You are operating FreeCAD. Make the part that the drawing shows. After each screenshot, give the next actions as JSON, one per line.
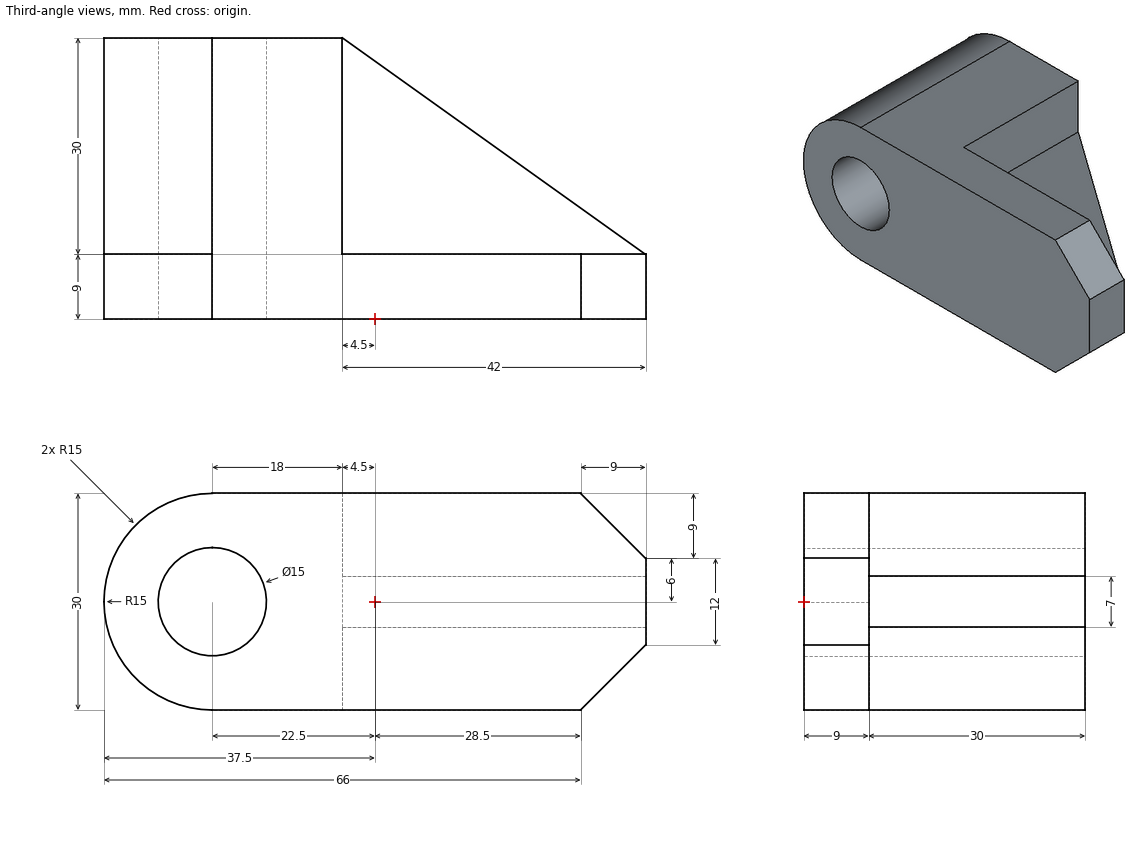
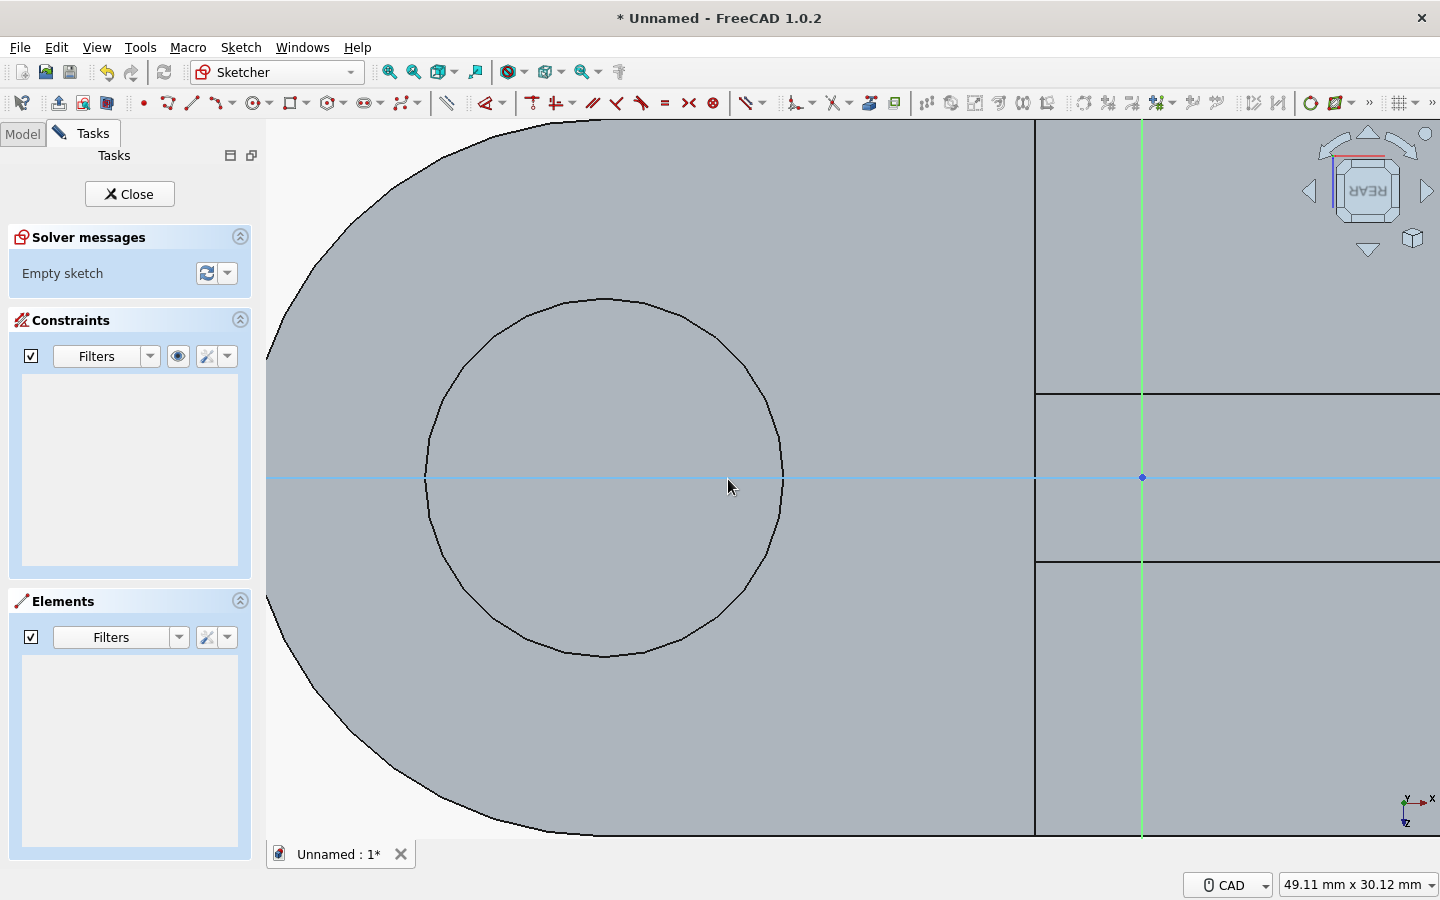
{"action": "left_click", "coordinate": [254, 104]}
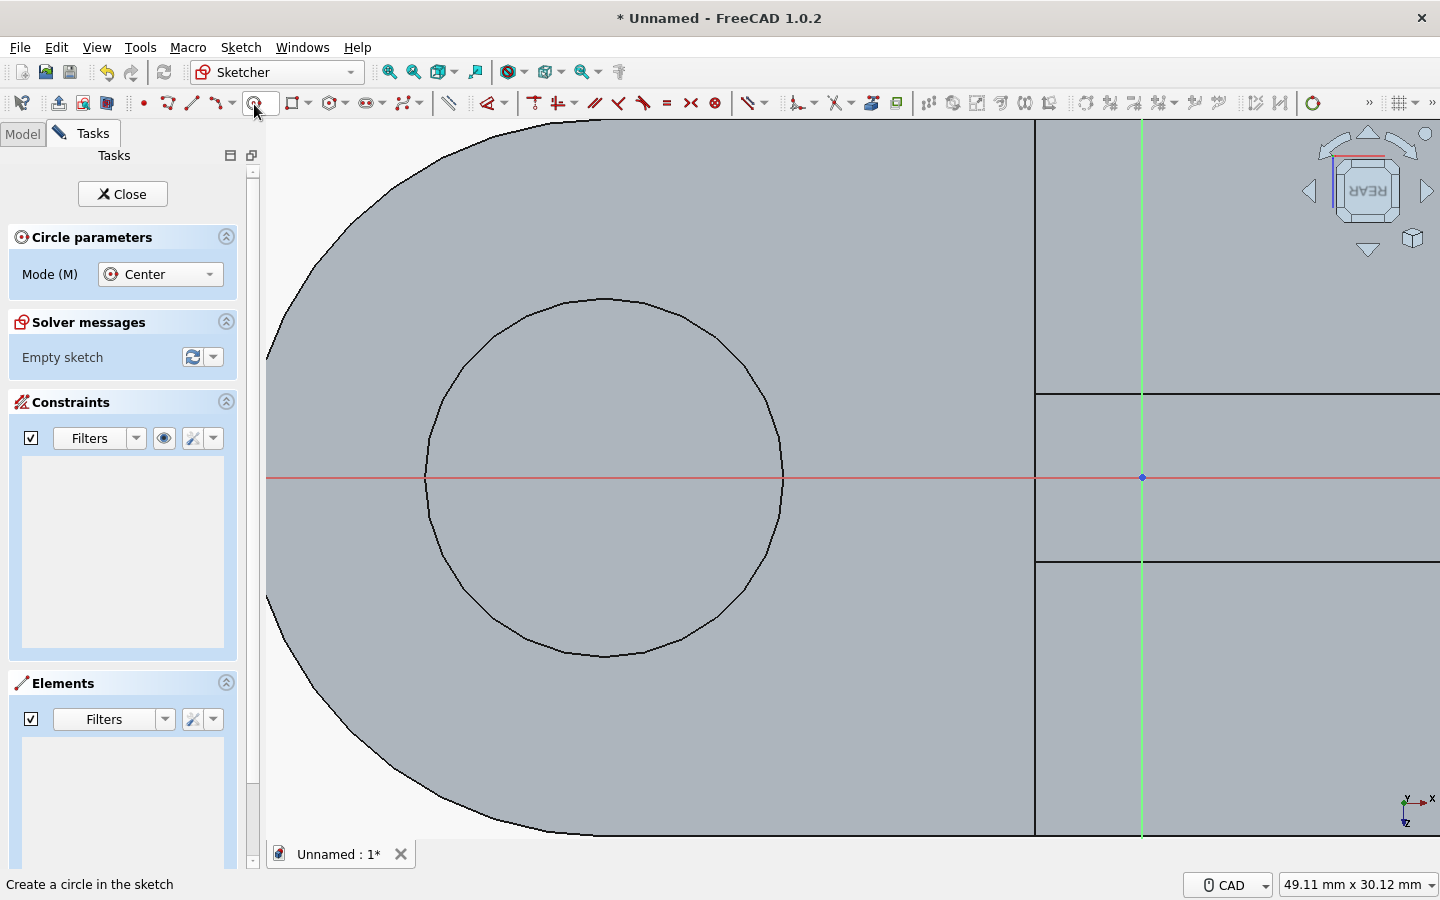
{"action": "left_click", "coordinate": [604, 478]}
{"action": "left_click", "coordinate": [731, 351]}
{"action": "key", "text": "Escape"}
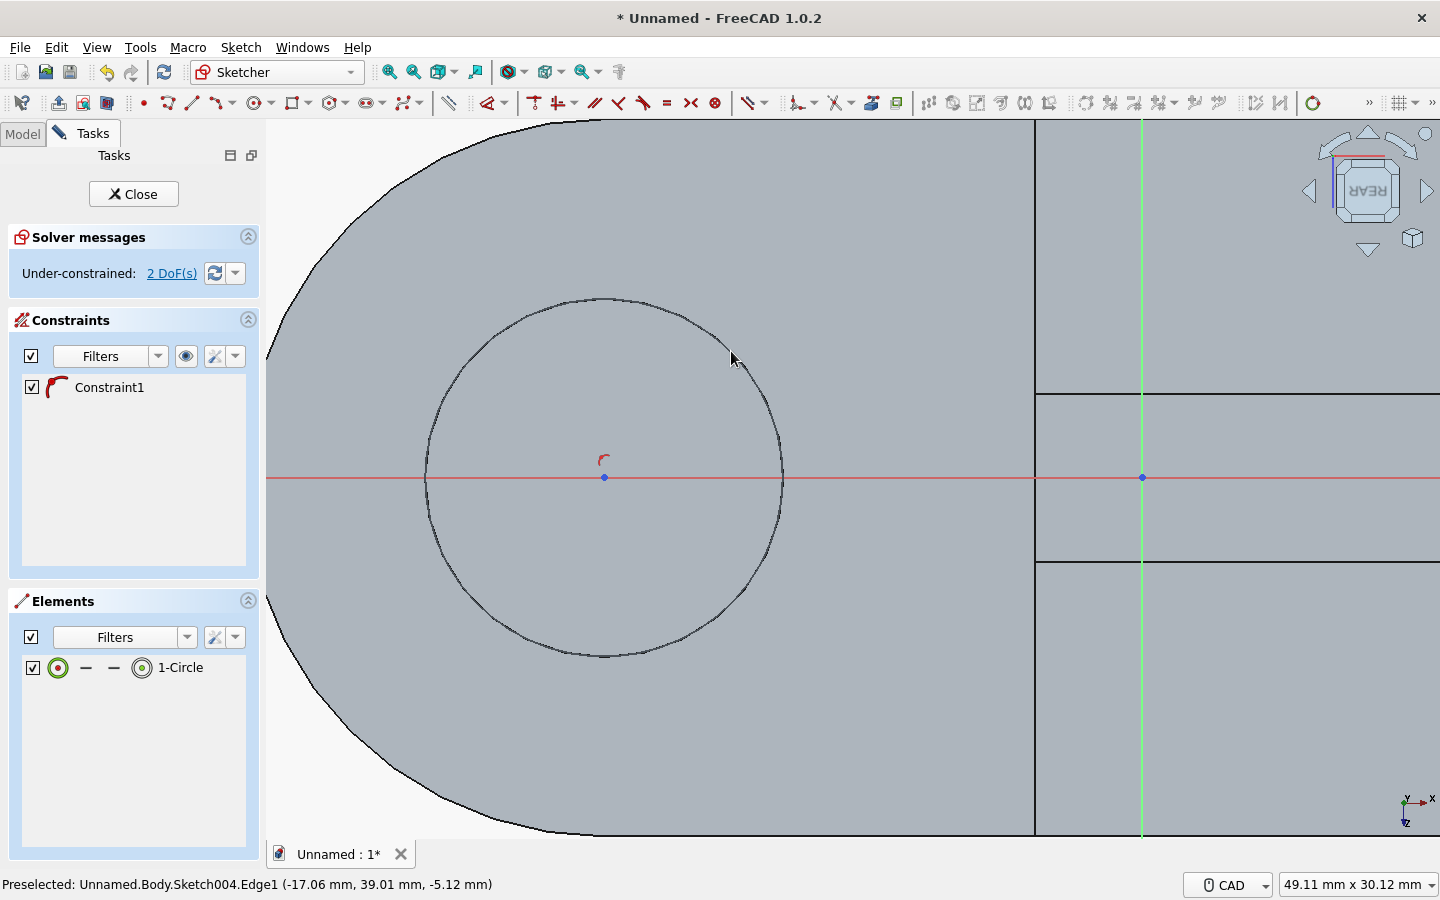
{"action": "key", "text": "d"}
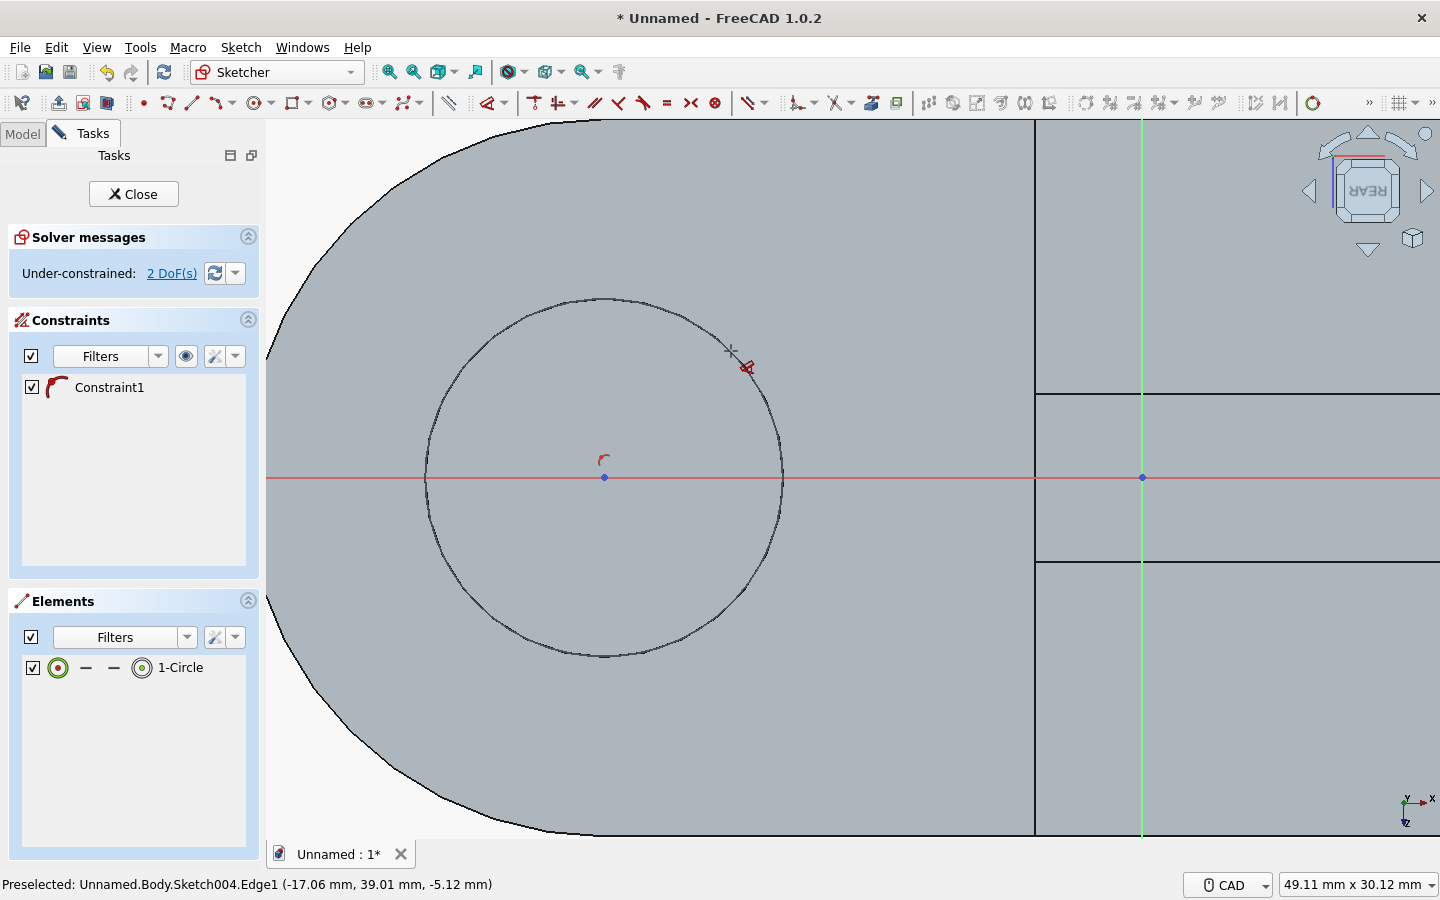
{"action": "left_click", "coordinate": [730, 351]}
{"action": "left_click", "coordinate": [753, 328]}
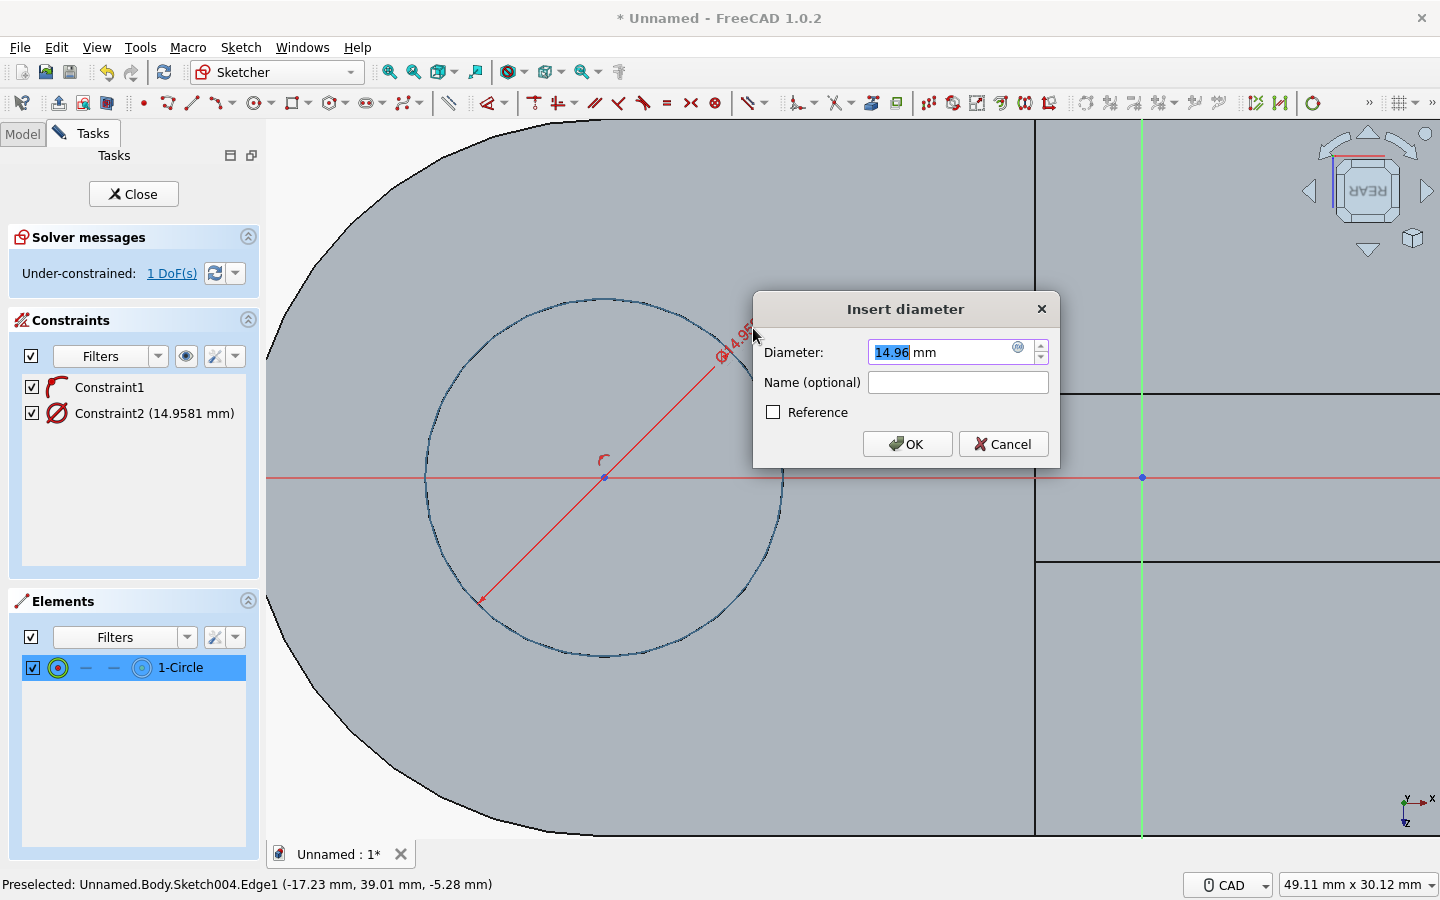
{"action": "type", "text": "15"}
{"action": "key", "text": "Return"}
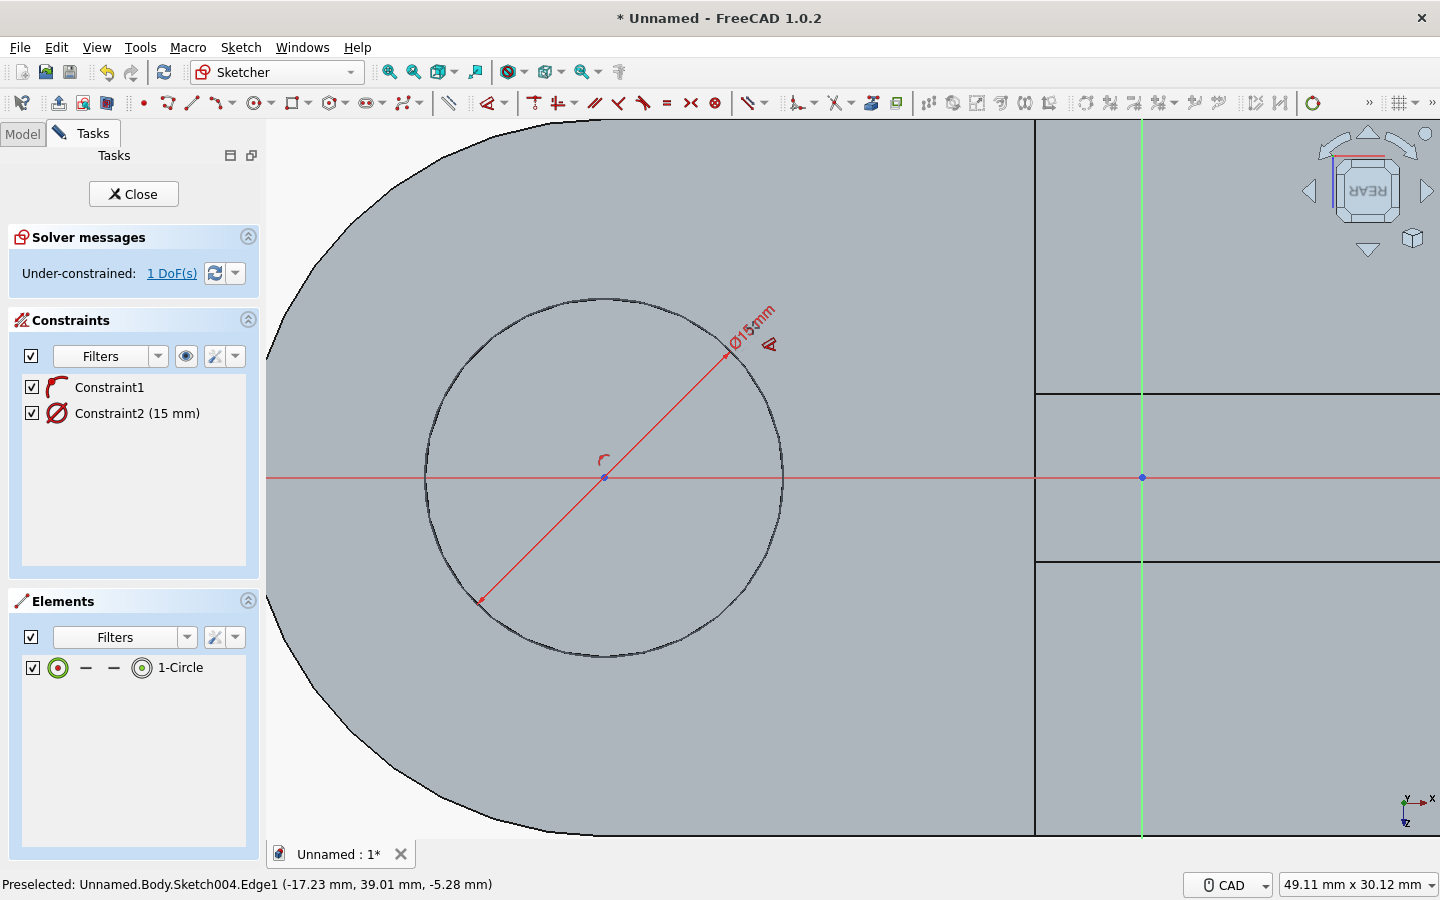
{"action": "left_click", "coordinate": [604, 478]}
{"action": "left_click", "coordinate": [873, 512]}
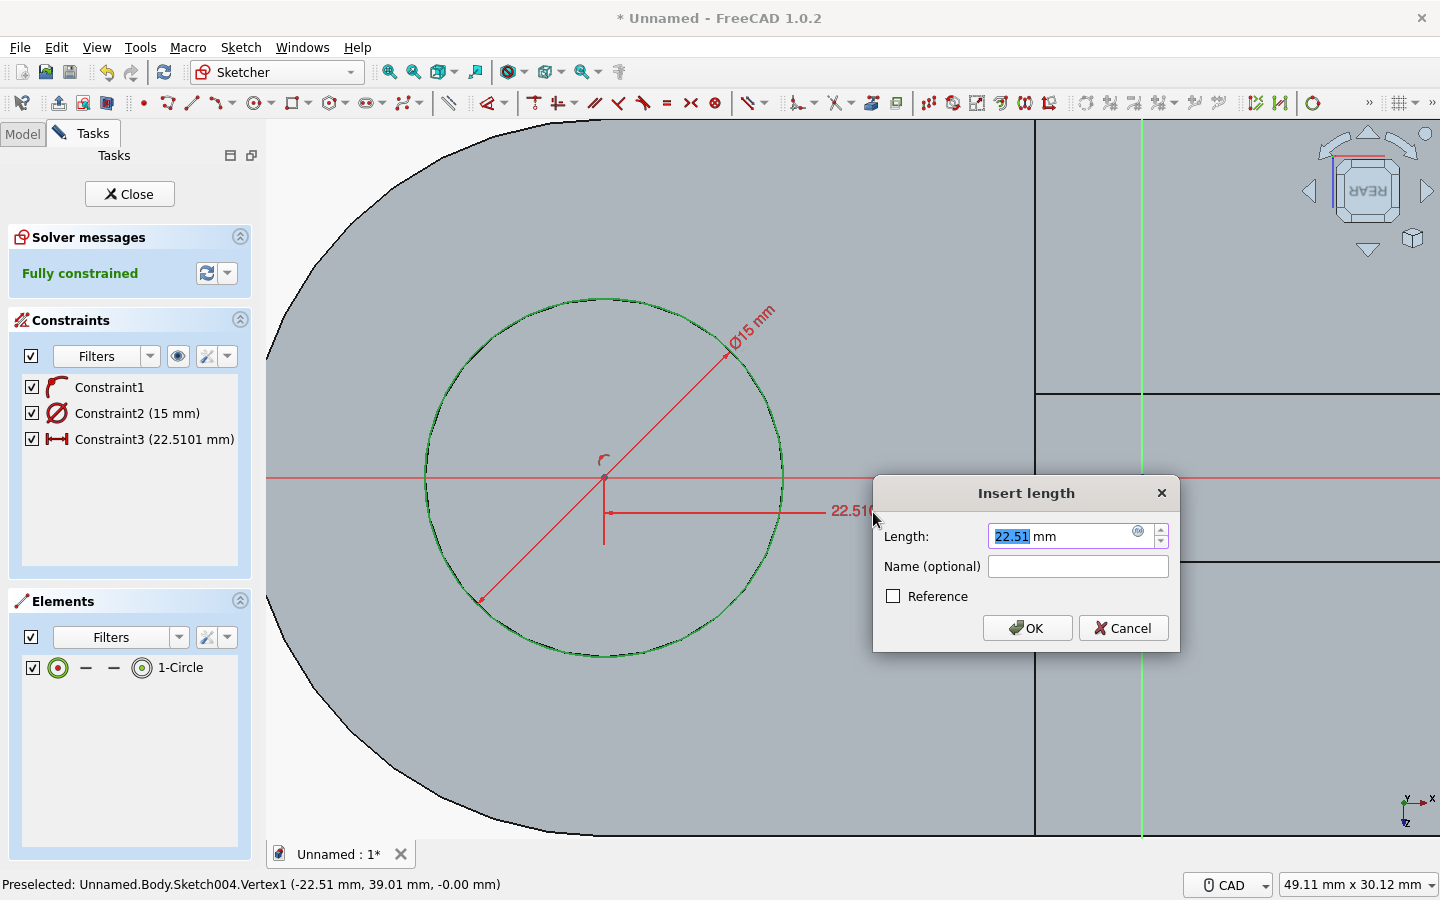
{"action": "type", "text": "22.5"}
{"action": "key", "text": "Return"}
{"action": "key", "text": "Escape"}